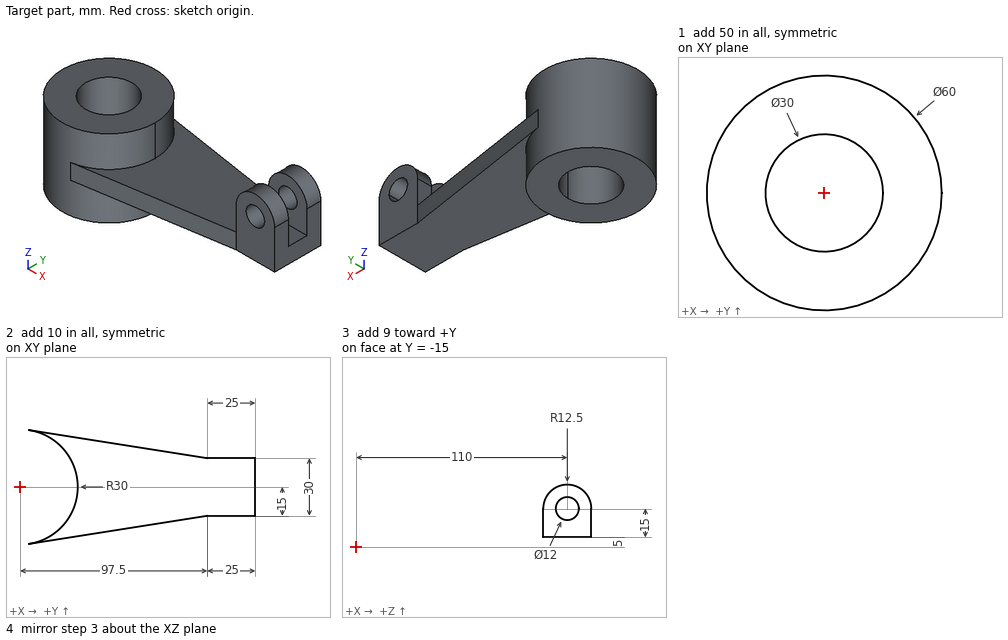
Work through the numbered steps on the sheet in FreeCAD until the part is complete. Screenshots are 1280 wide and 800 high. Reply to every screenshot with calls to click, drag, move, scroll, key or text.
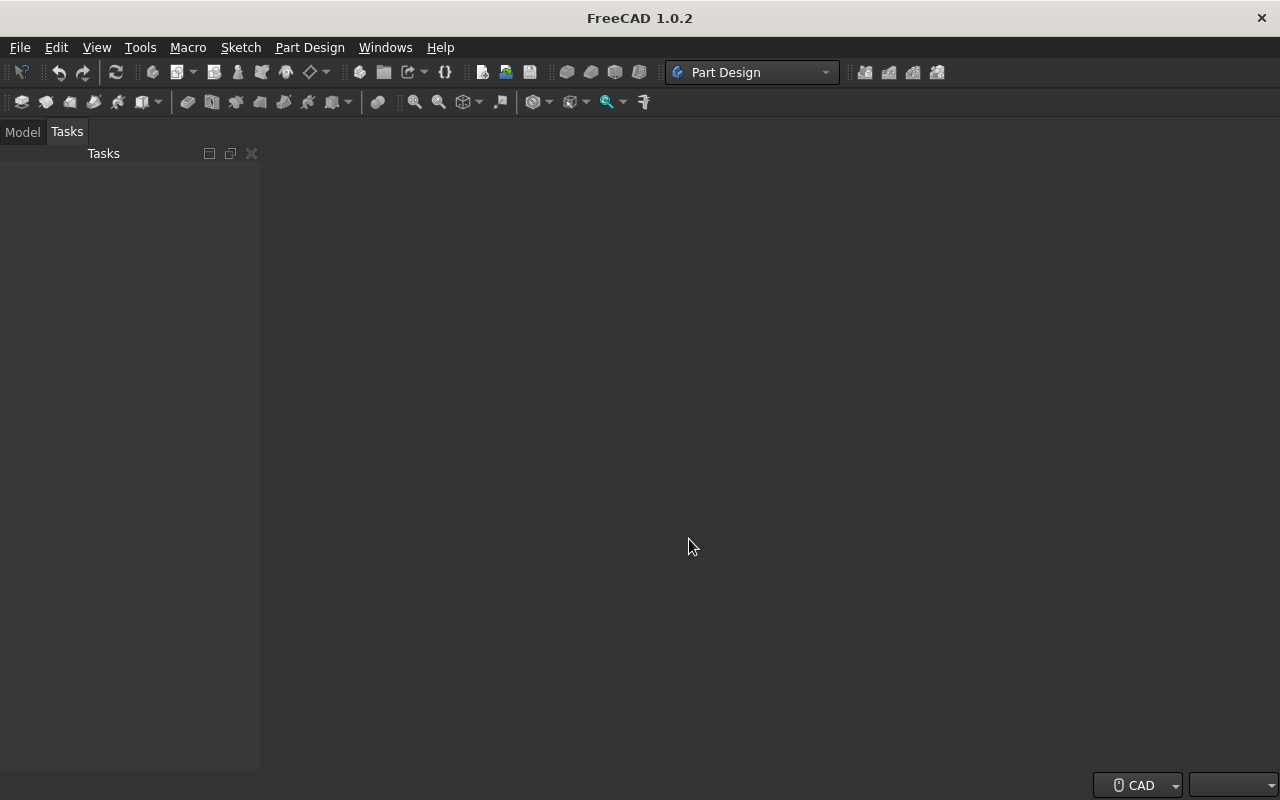
click(482, 72)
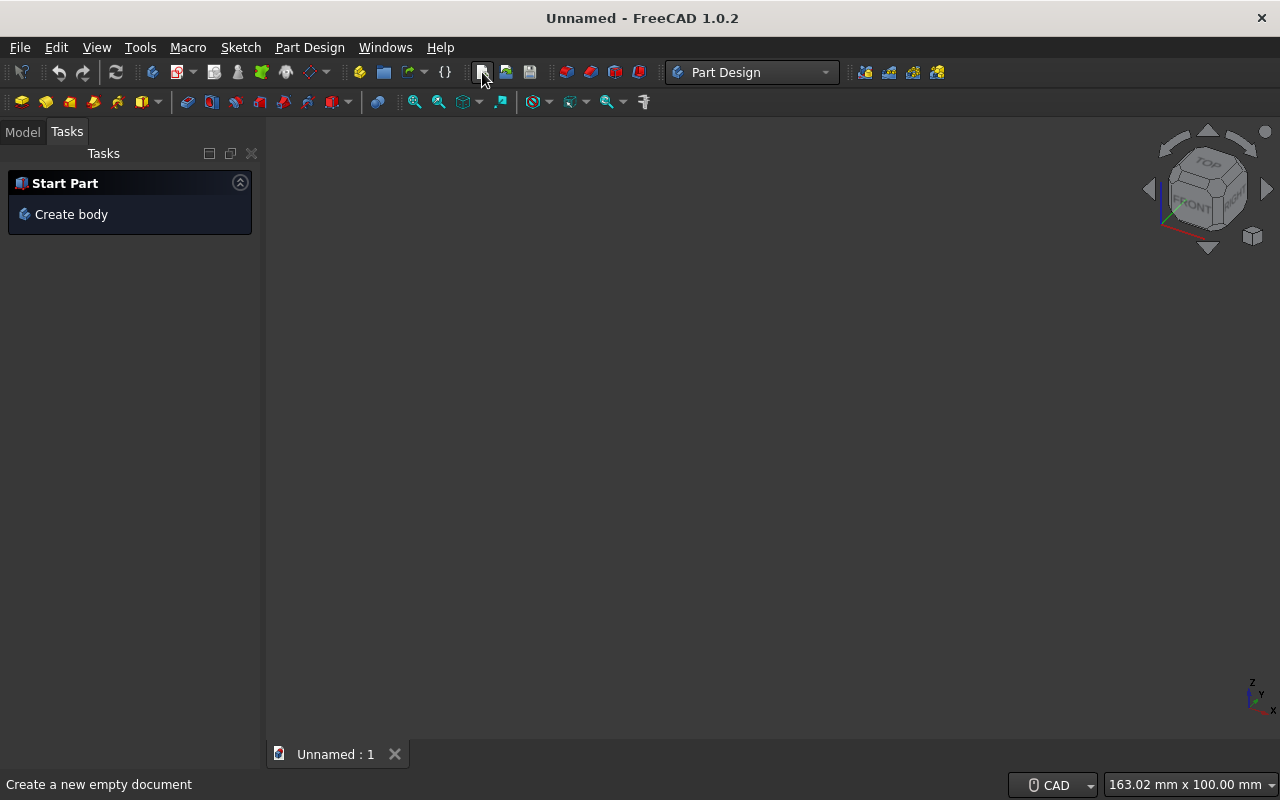
click(178, 72)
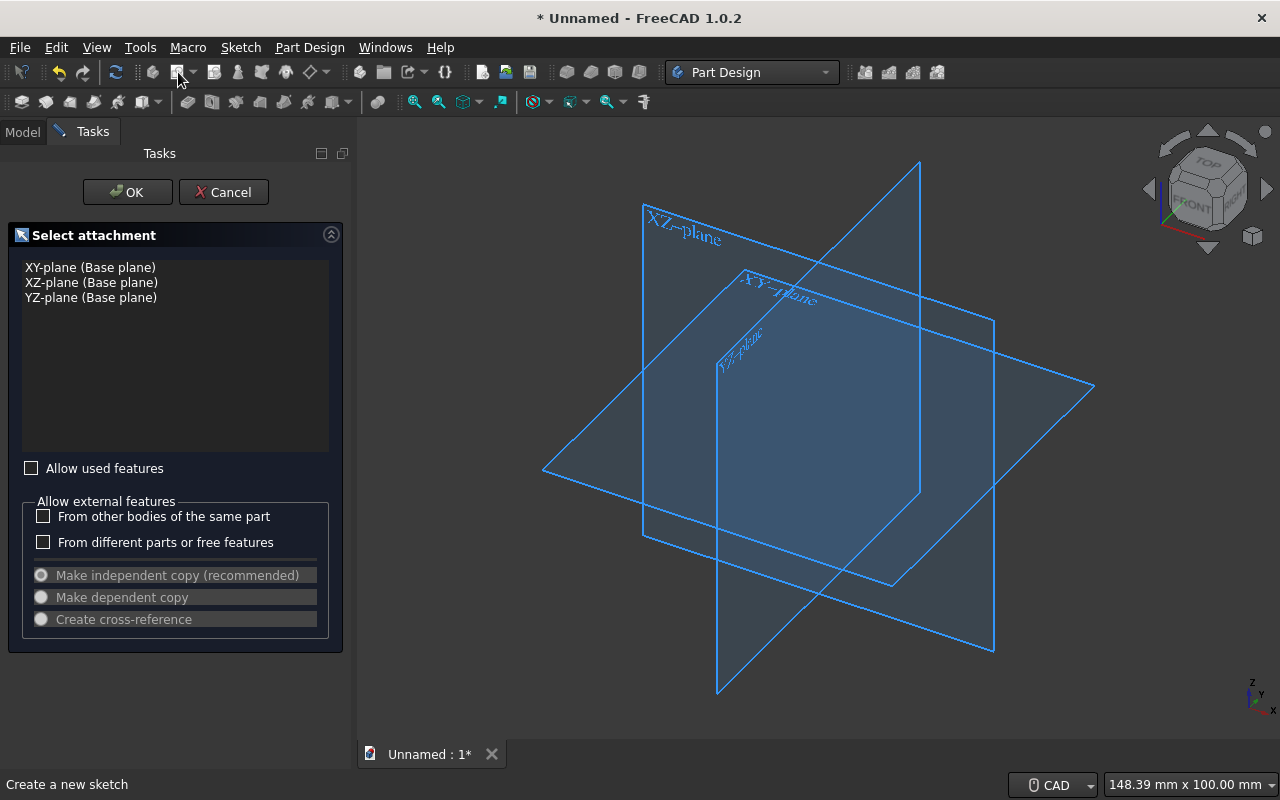
click(82, 268)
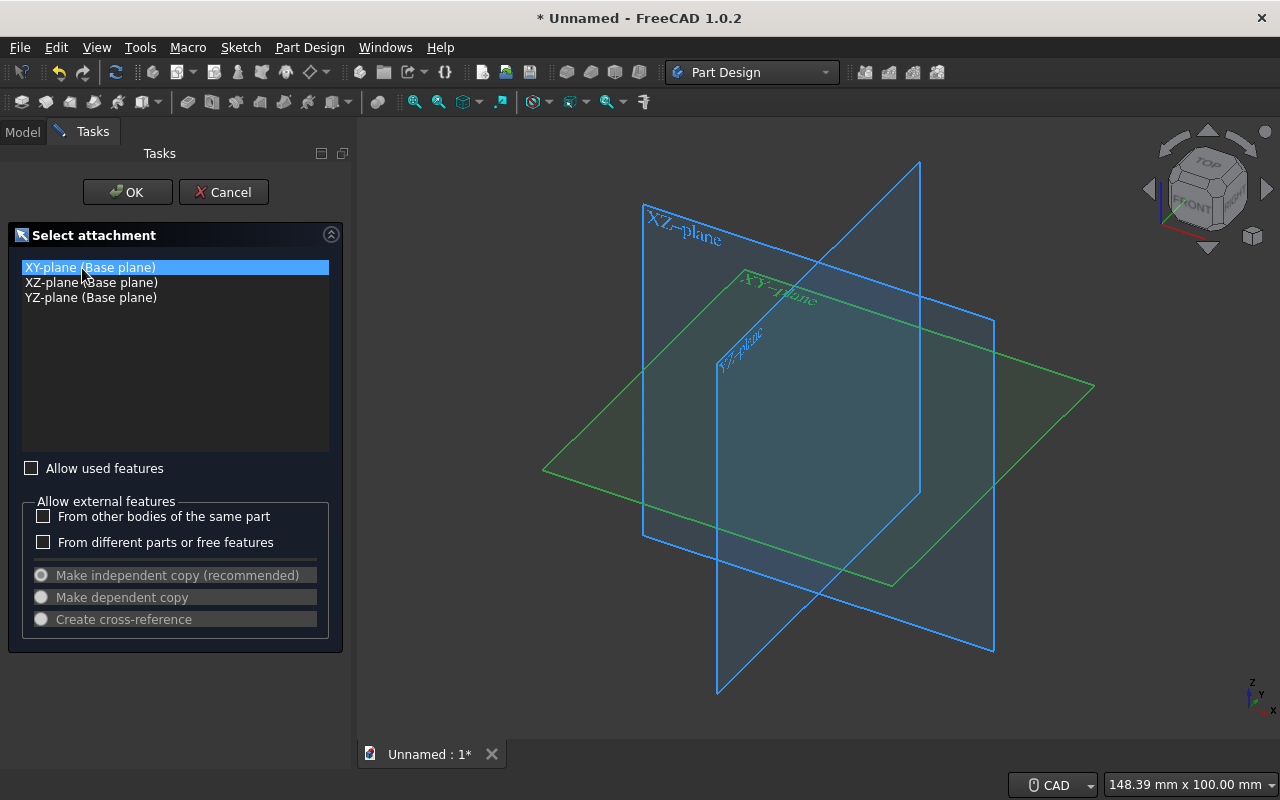
click(128, 192)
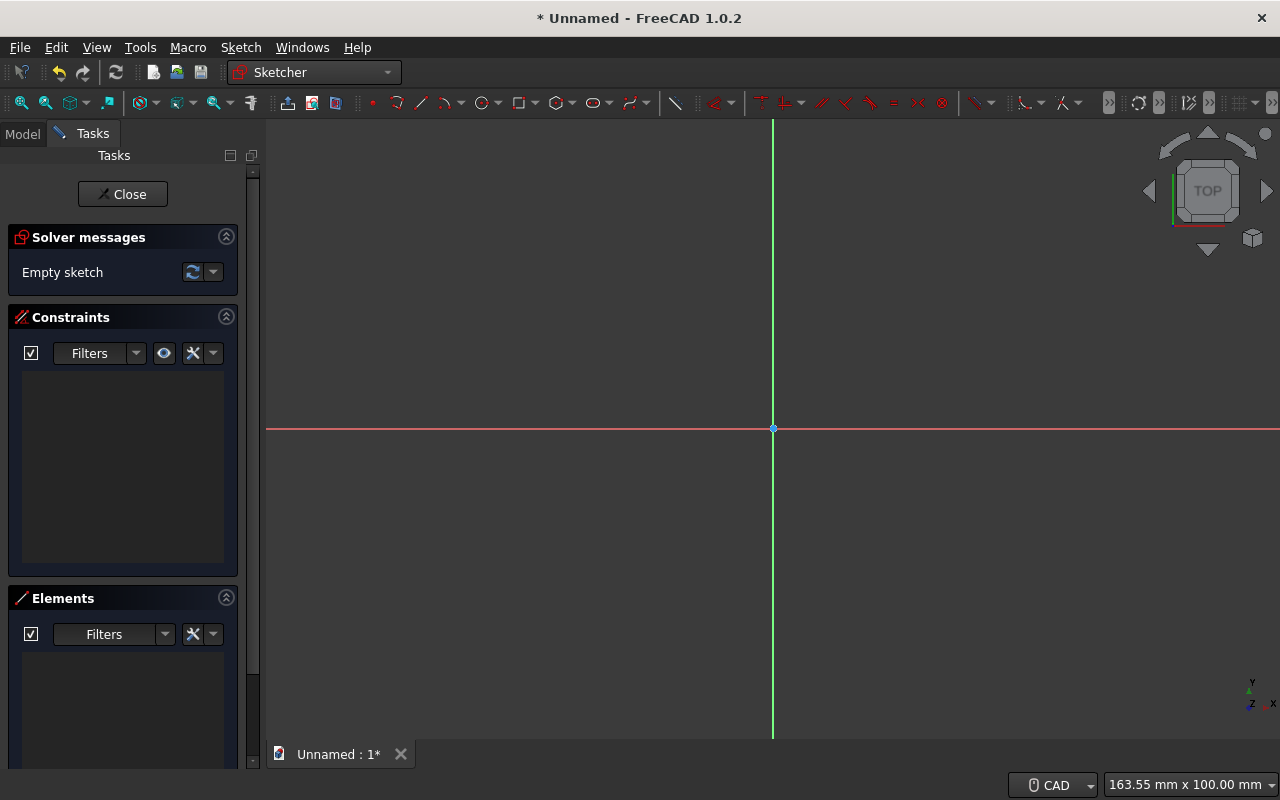
click(482, 104)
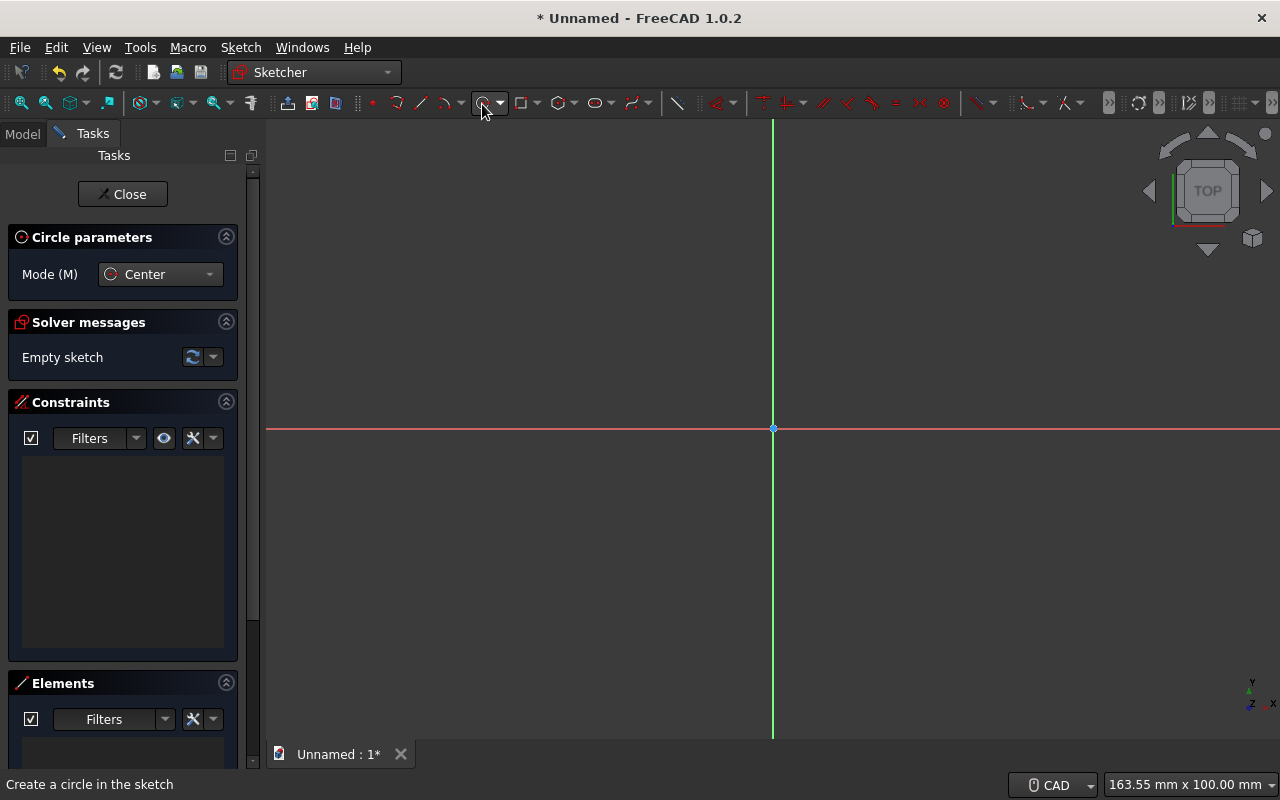
click(773, 429)
click(905, 297)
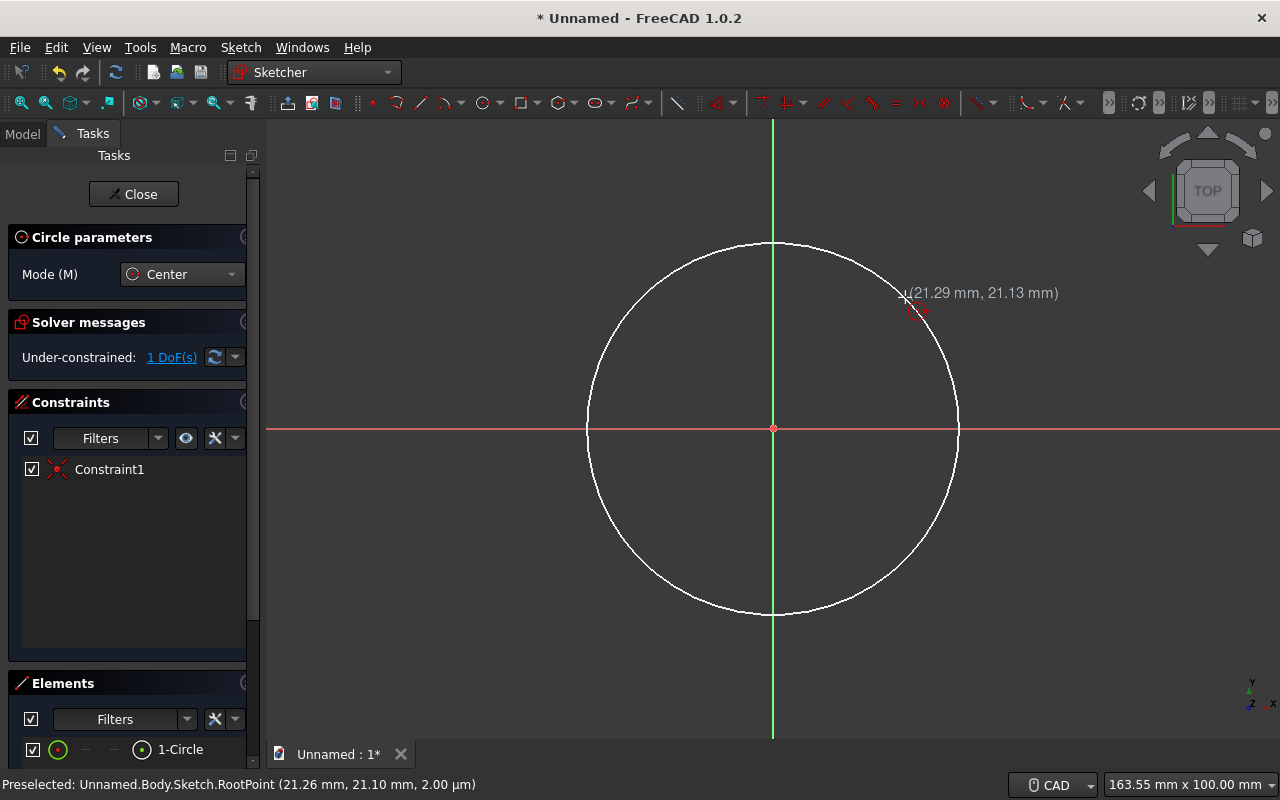
click(773, 429)
click(839, 363)
key(Escape)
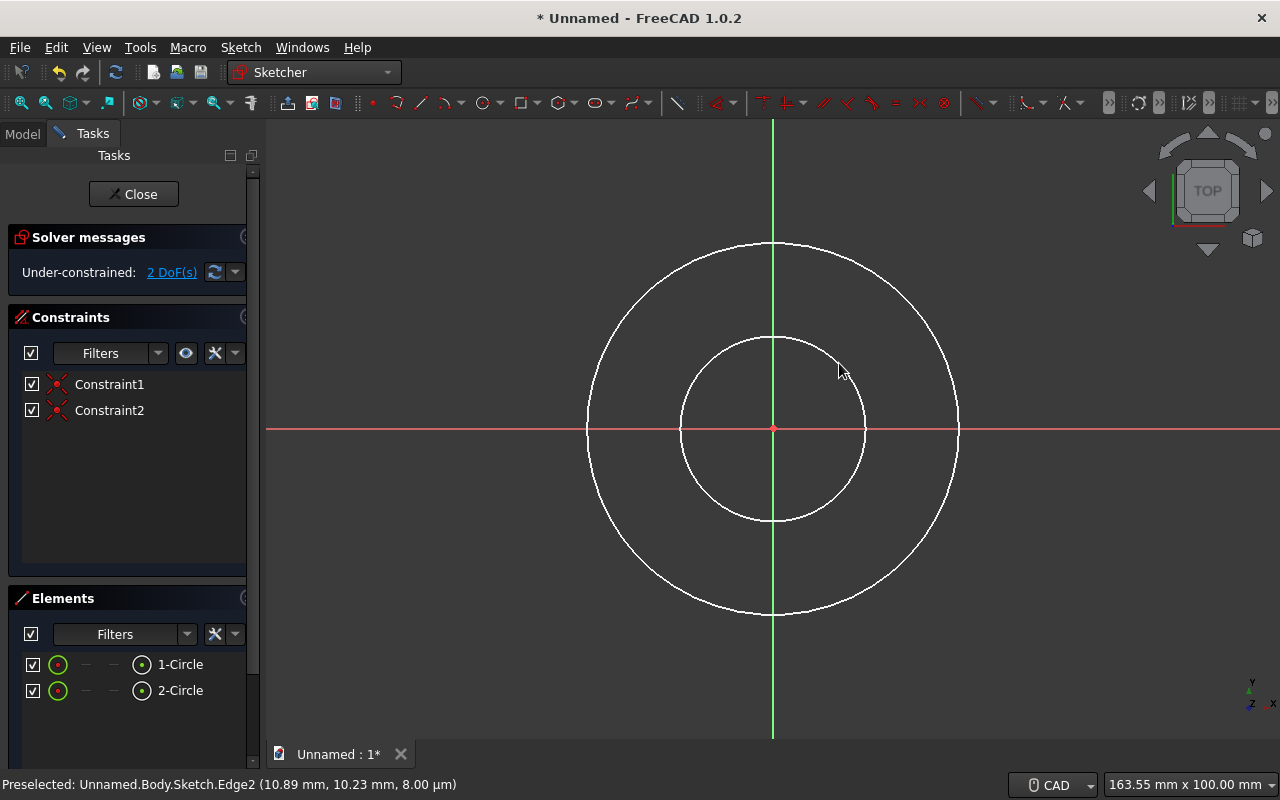
click(716, 104)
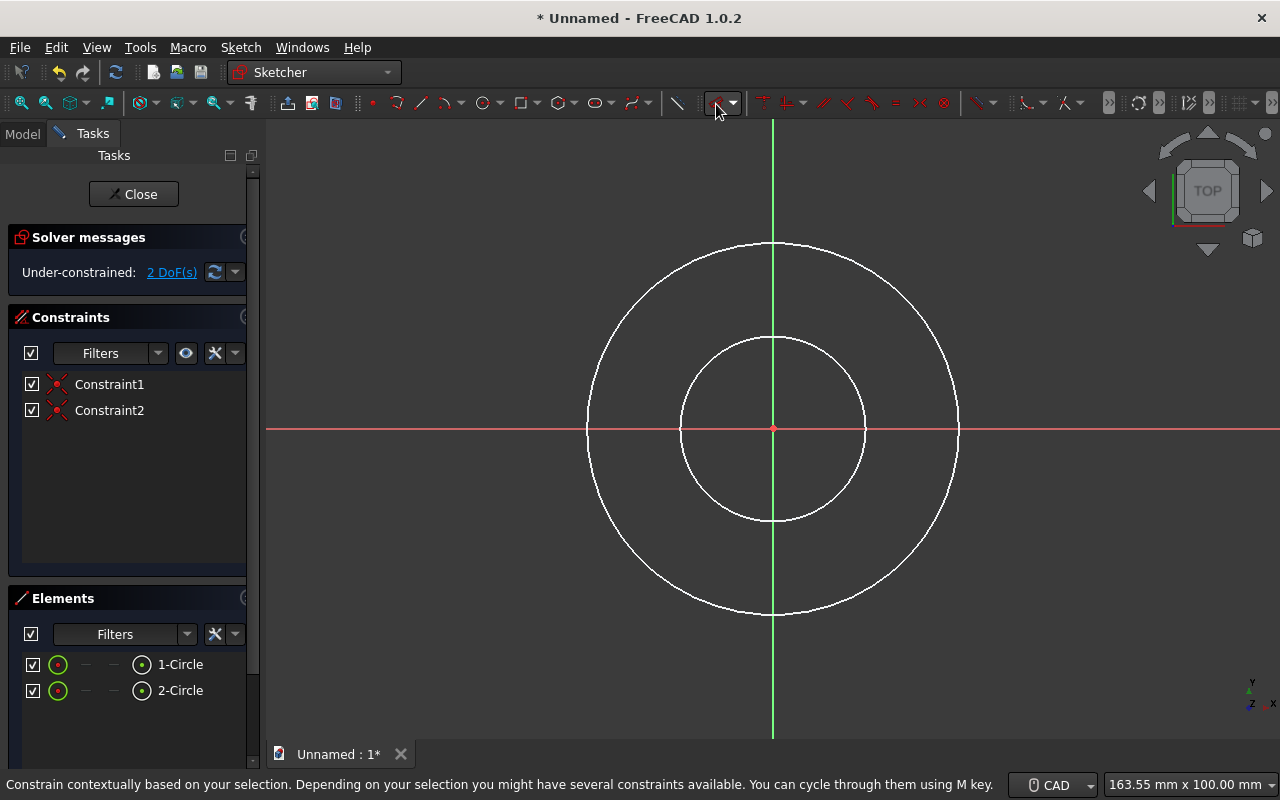
click(904, 297)
click(927, 274)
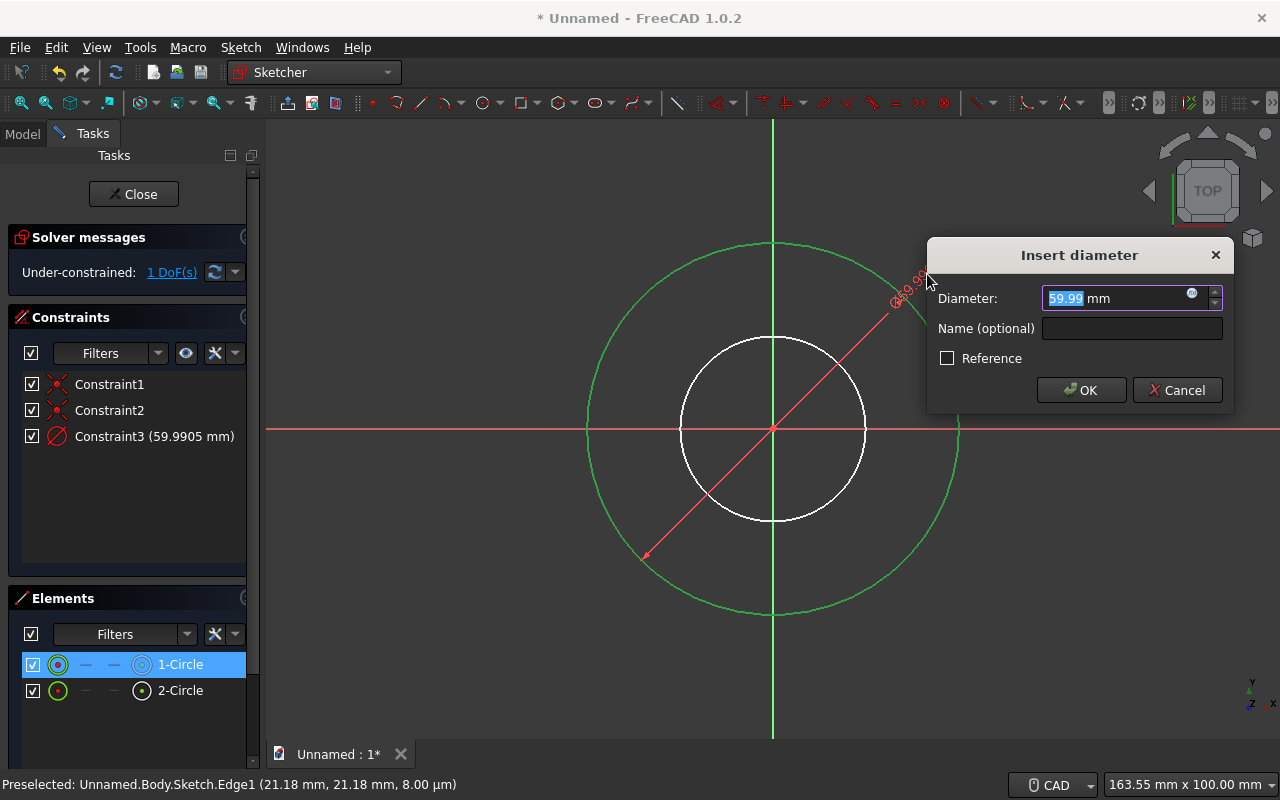
text(60)
key(Return)